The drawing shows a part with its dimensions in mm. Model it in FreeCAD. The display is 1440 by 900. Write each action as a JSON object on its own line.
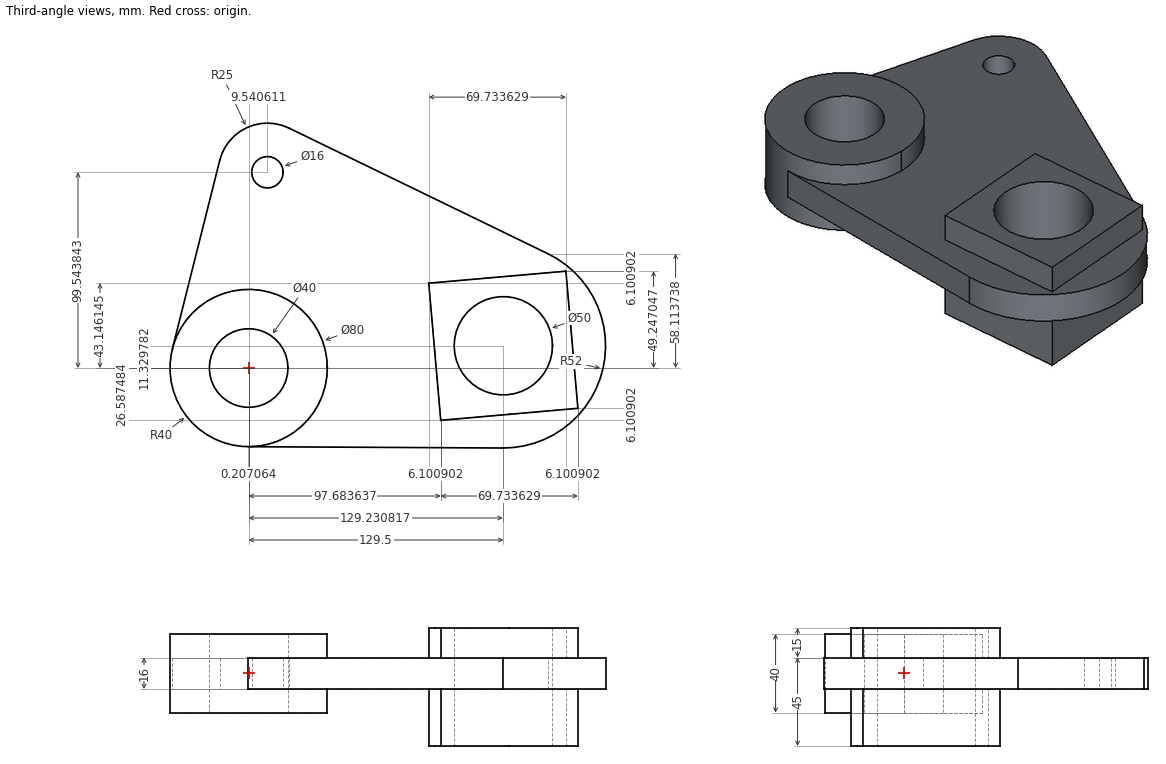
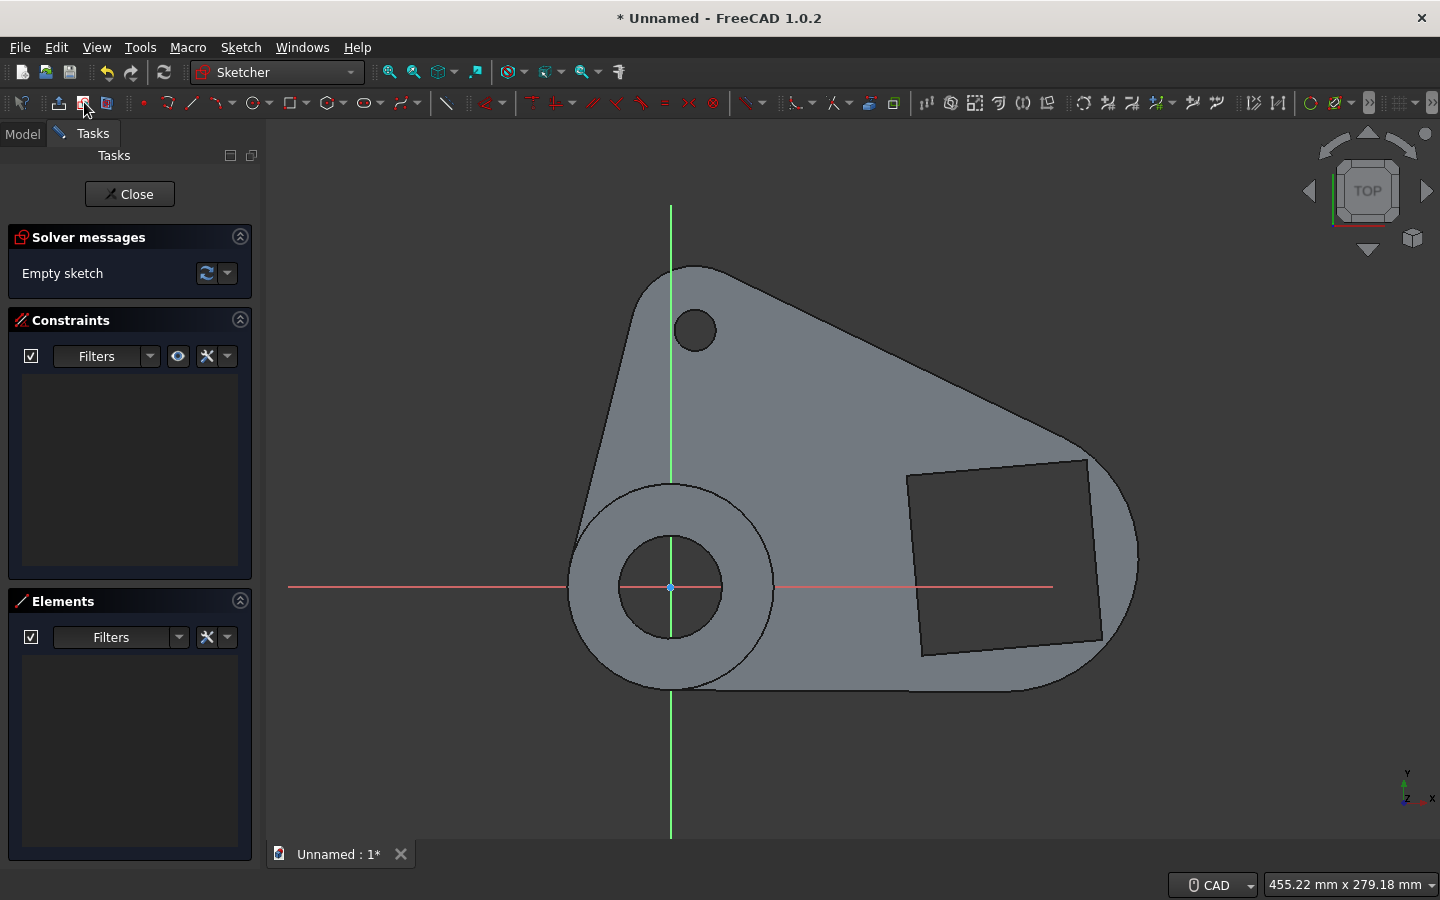
{"action": "scroll", "coordinate": [1094, 718], "scroll_direction": "up", "scroll_amount": 2}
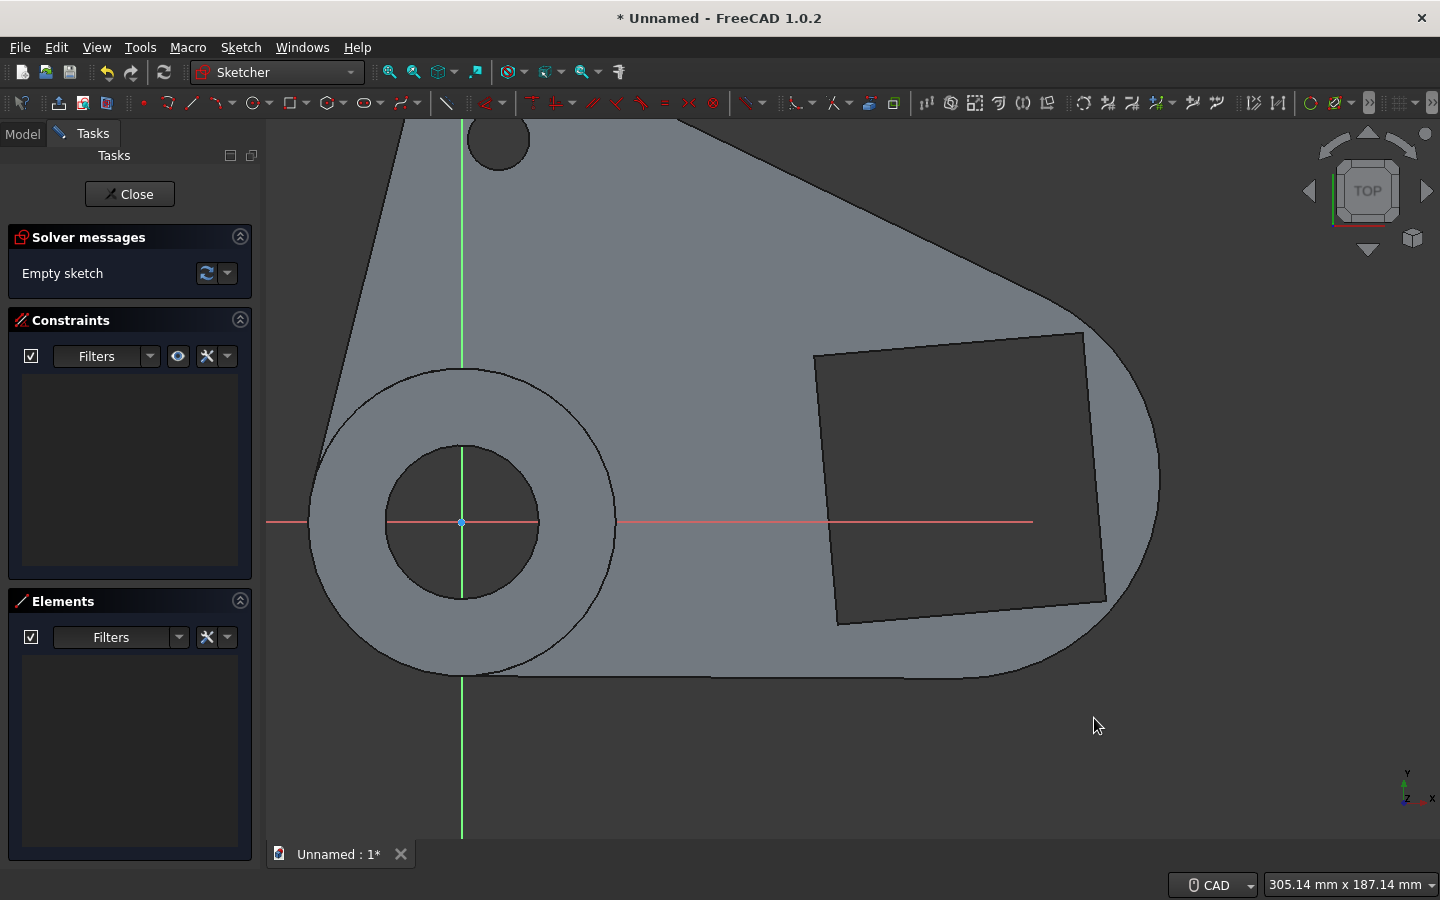
{"action": "left_click", "coordinate": [168, 104]}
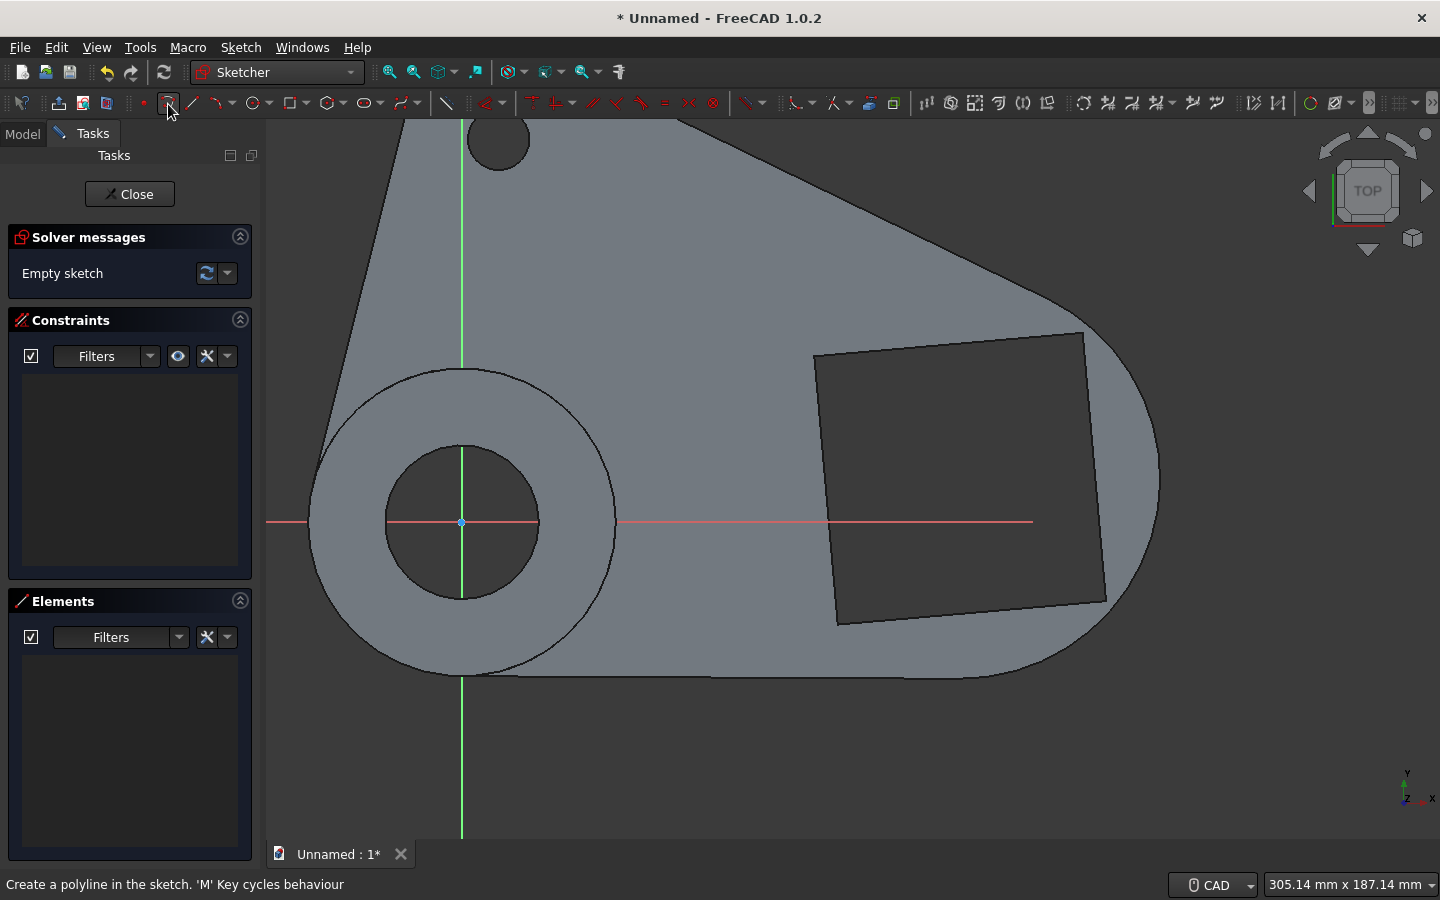
{"action": "left_click", "coordinate": [838, 625]}
{"action": "left_click", "coordinate": [1106, 601]}
{"action": "left_click", "coordinate": [1083, 333]}
{"action": "left_click", "coordinate": [814, 356]}
{"action": "left_click", "coordinate": [838, 626]}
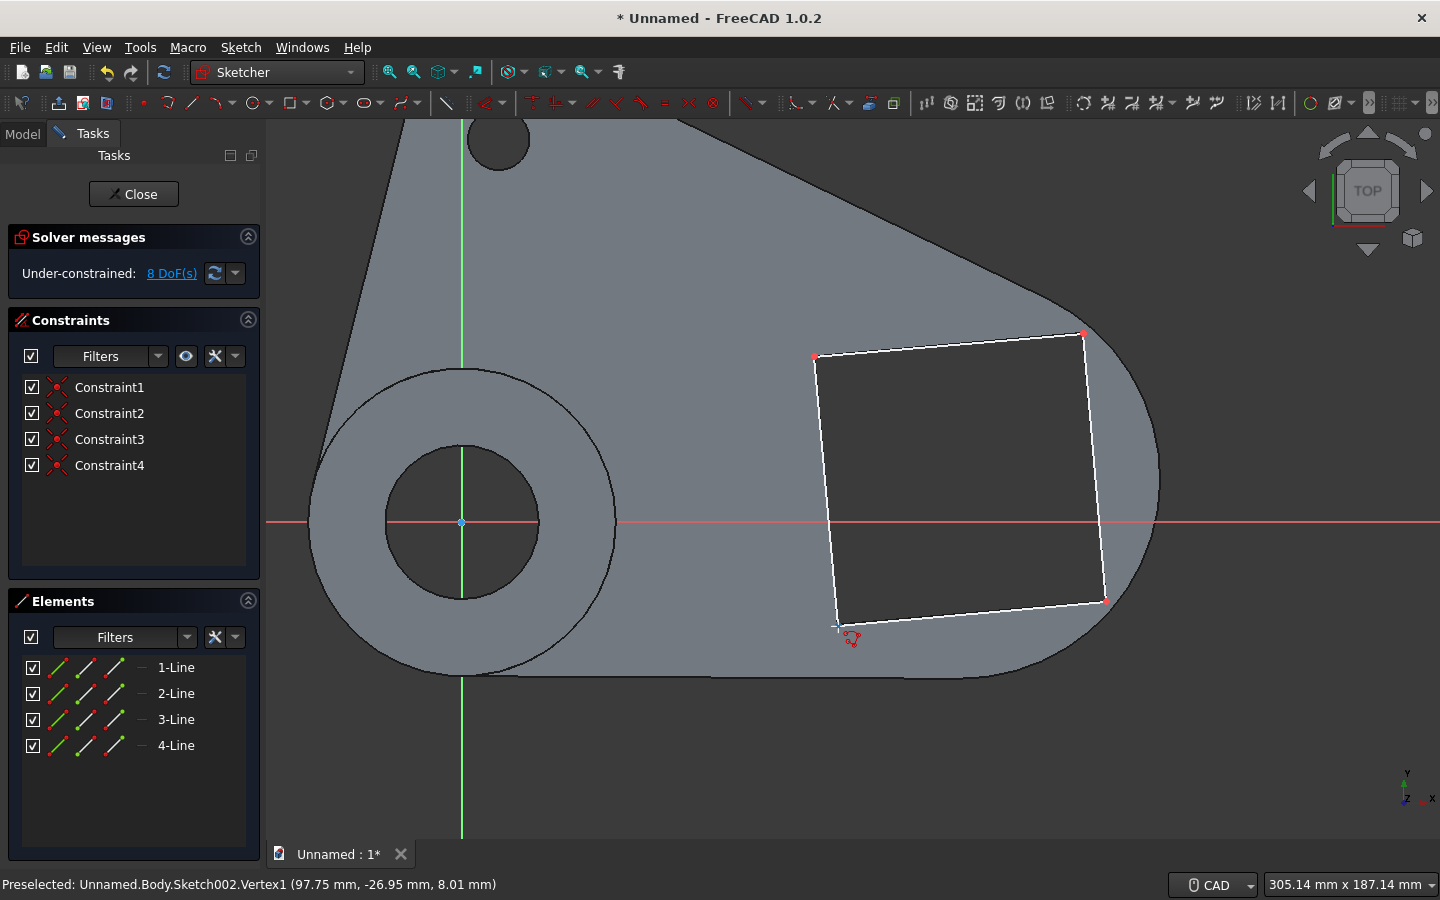
{"action": "key", "text": "g c"}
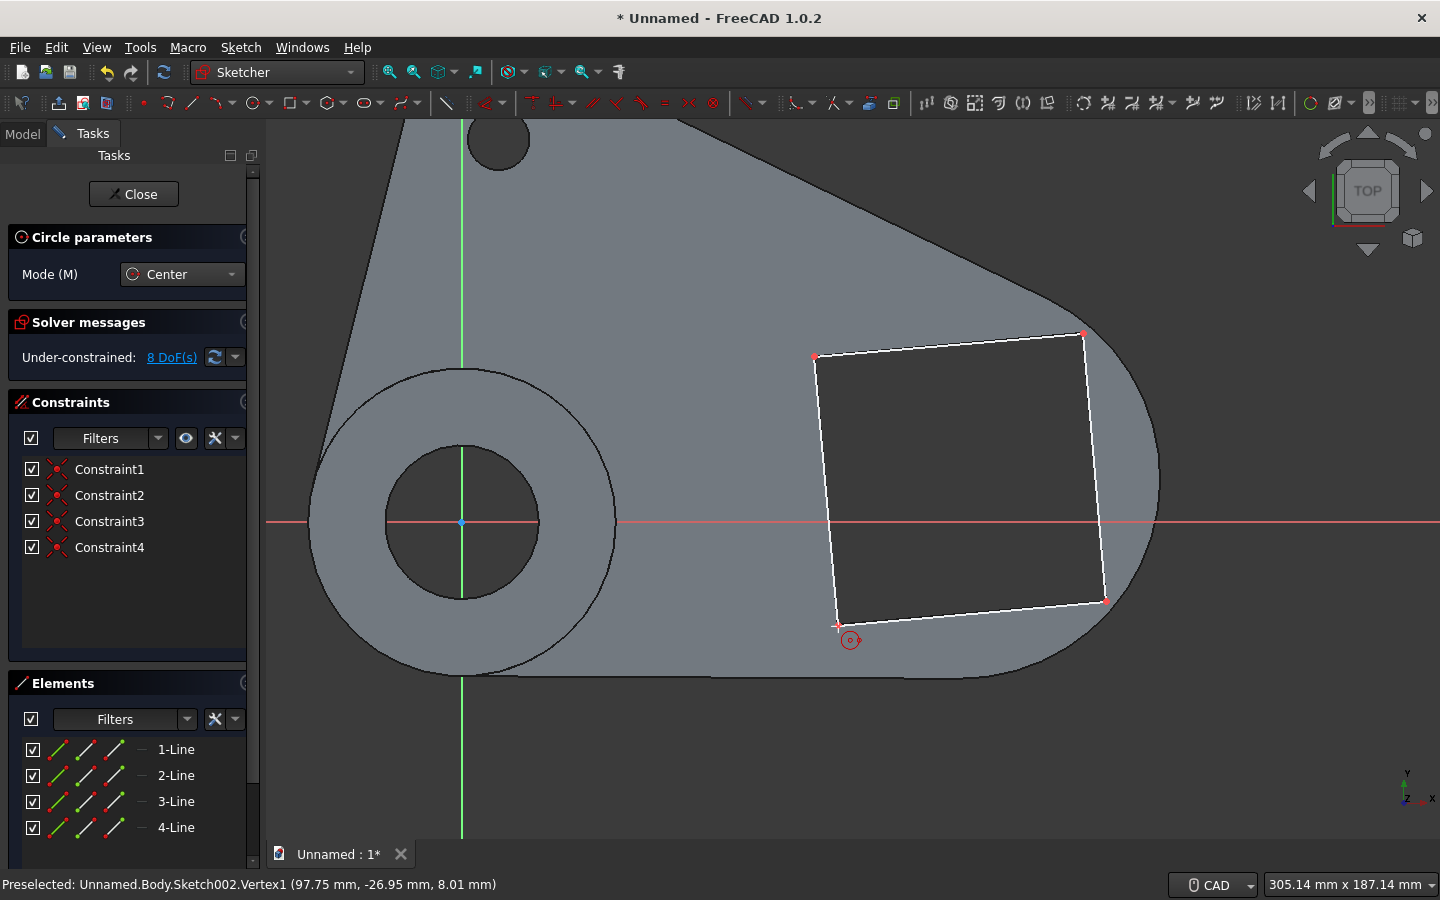
{"action": "left_click", "coordinate": [960, 479]}
{"action": "left_click", "coordinate": [1028, 411]}
{"action": "key", "text": "Escape"}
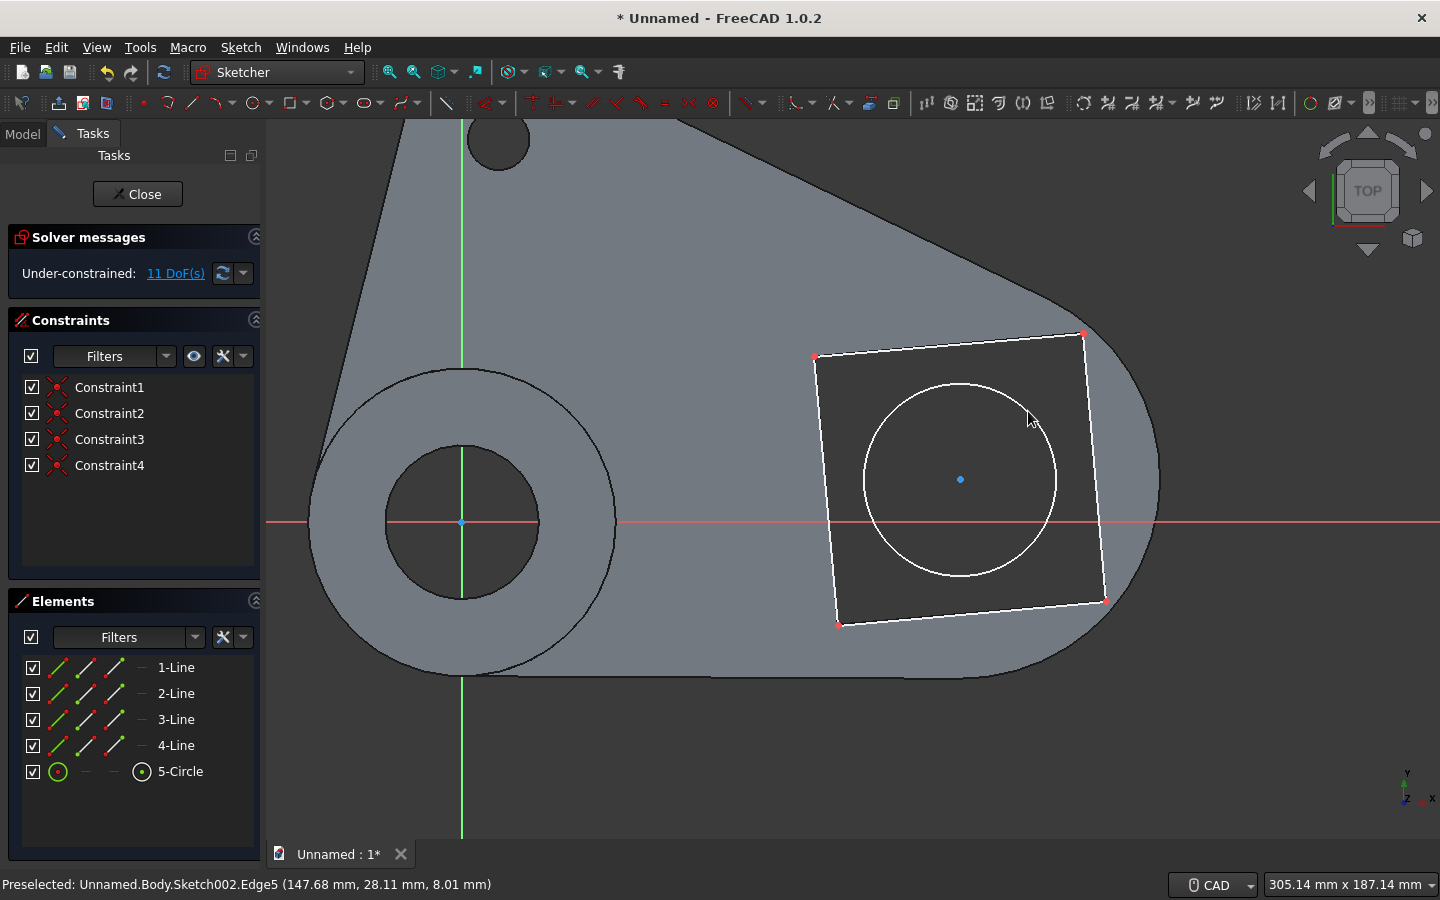
{"action": "left_click", "coordinate": [486, 104]}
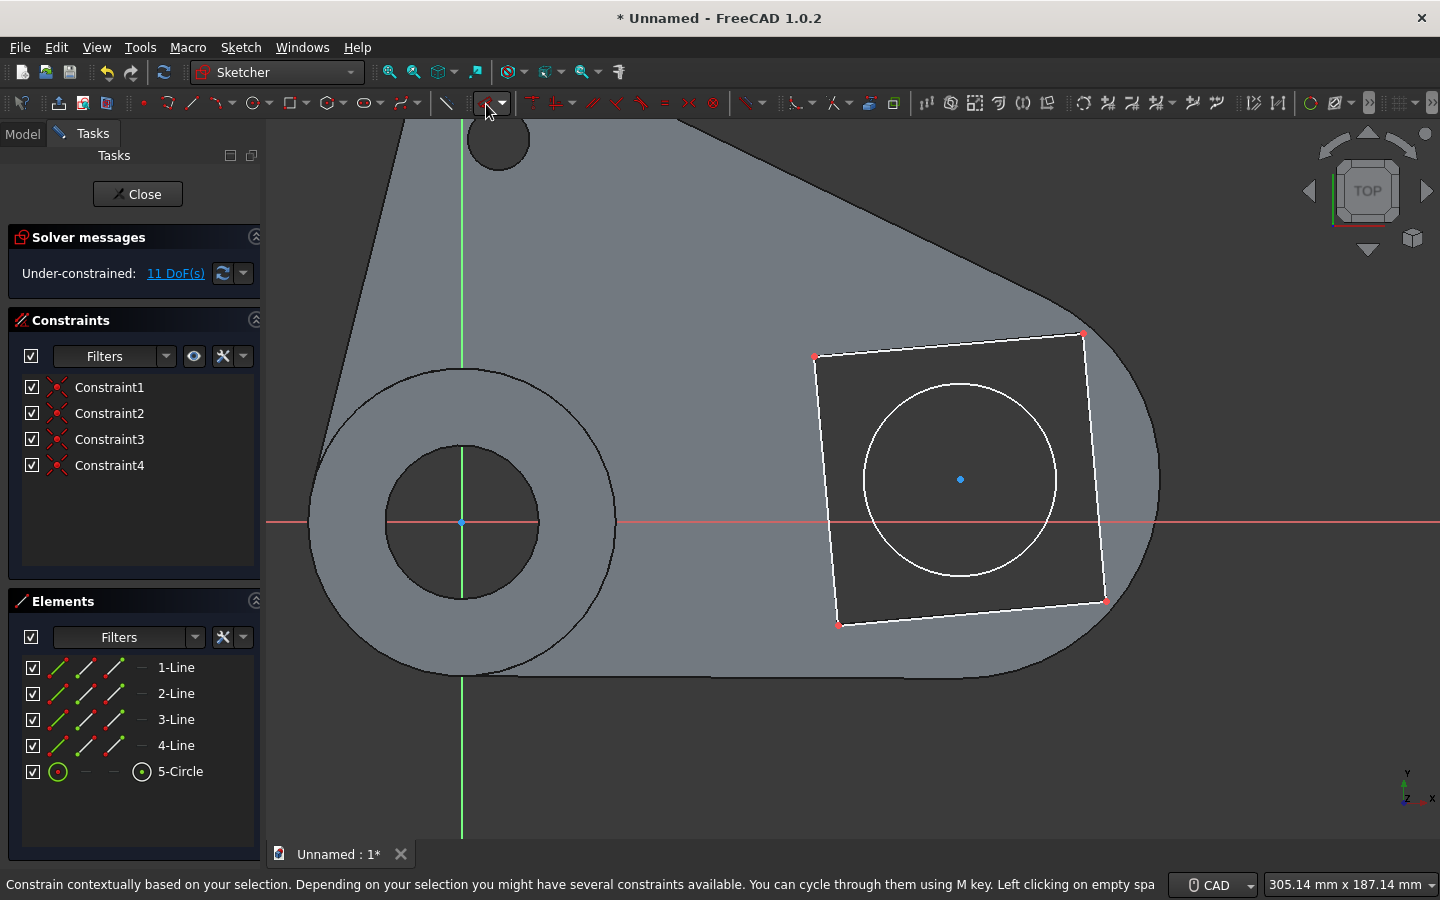
{"action": "left_click", "coordinate": [1028, 412]}
{"action": "left_click", "coordinate": [1051, 389]}